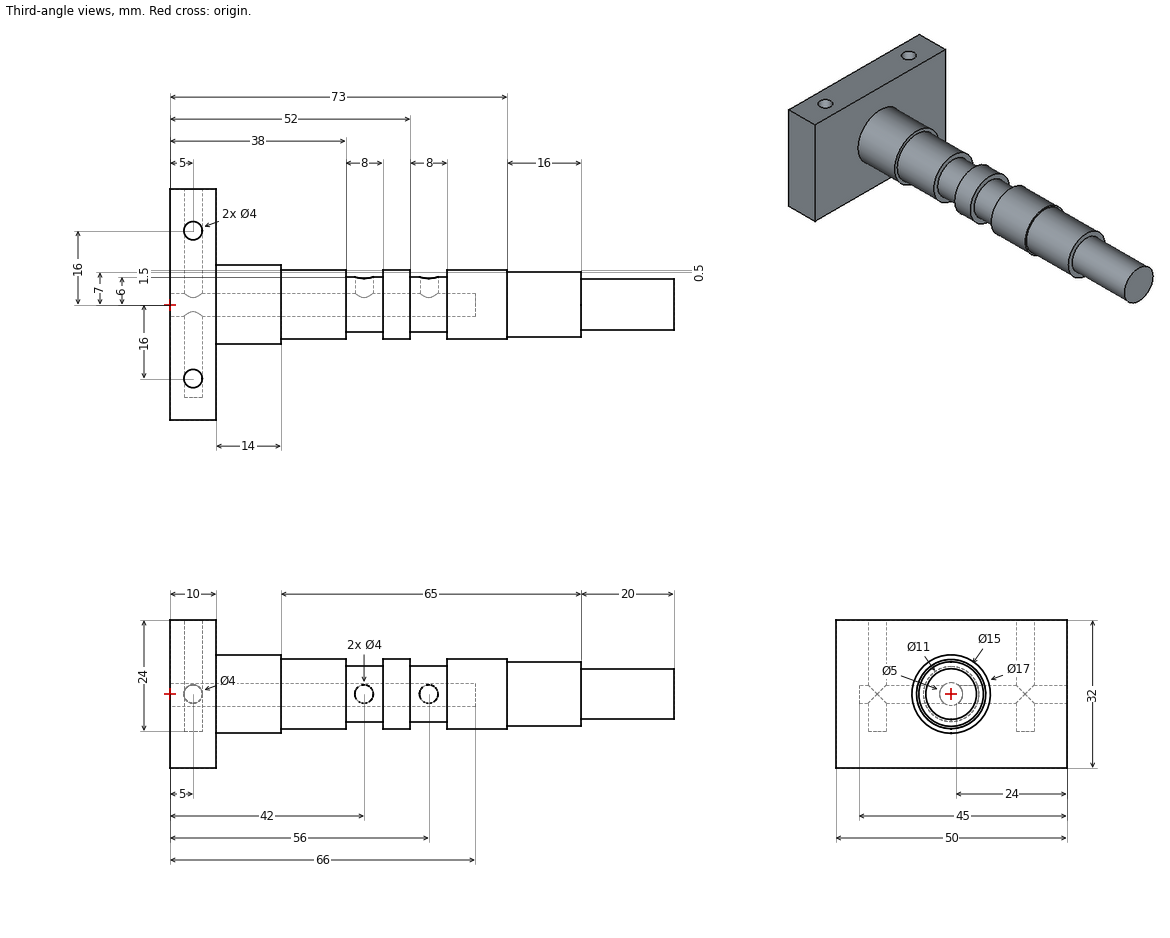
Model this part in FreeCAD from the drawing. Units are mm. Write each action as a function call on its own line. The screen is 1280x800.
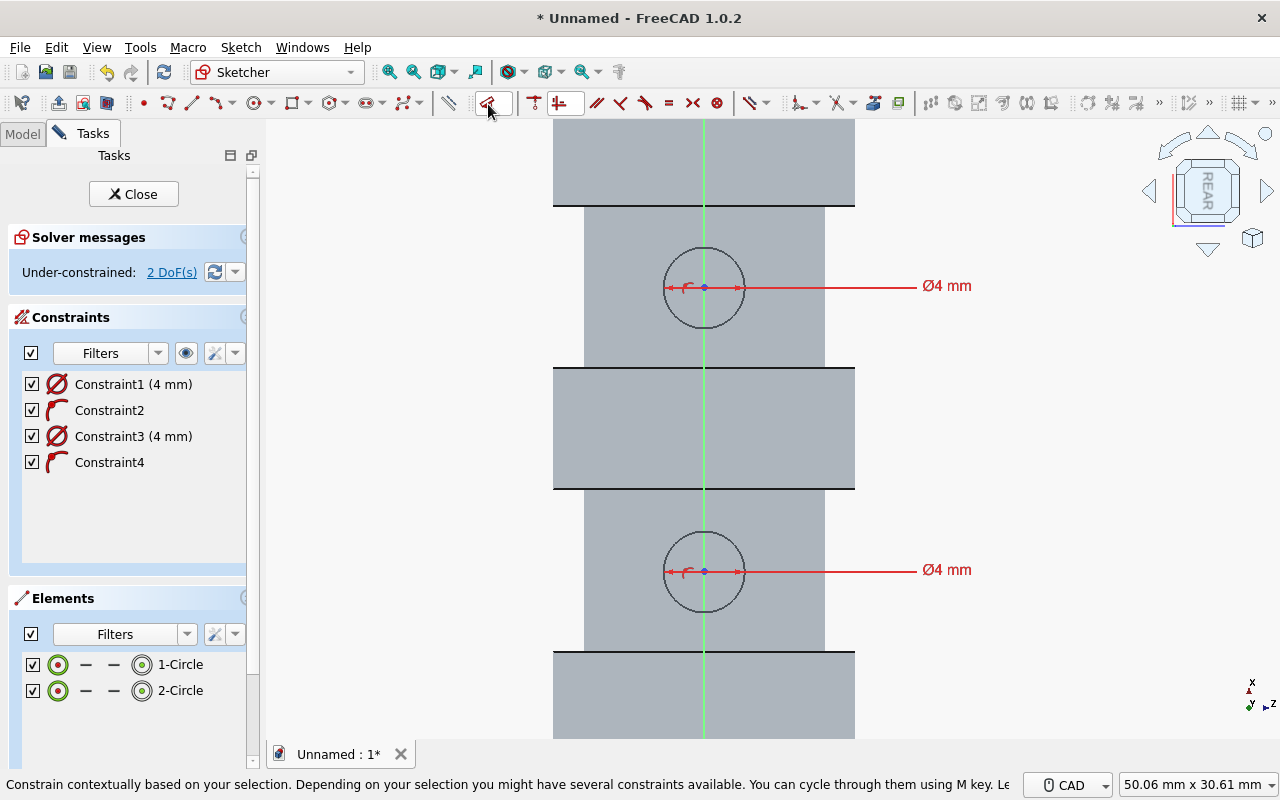
click(704, 572)
click(738, 642)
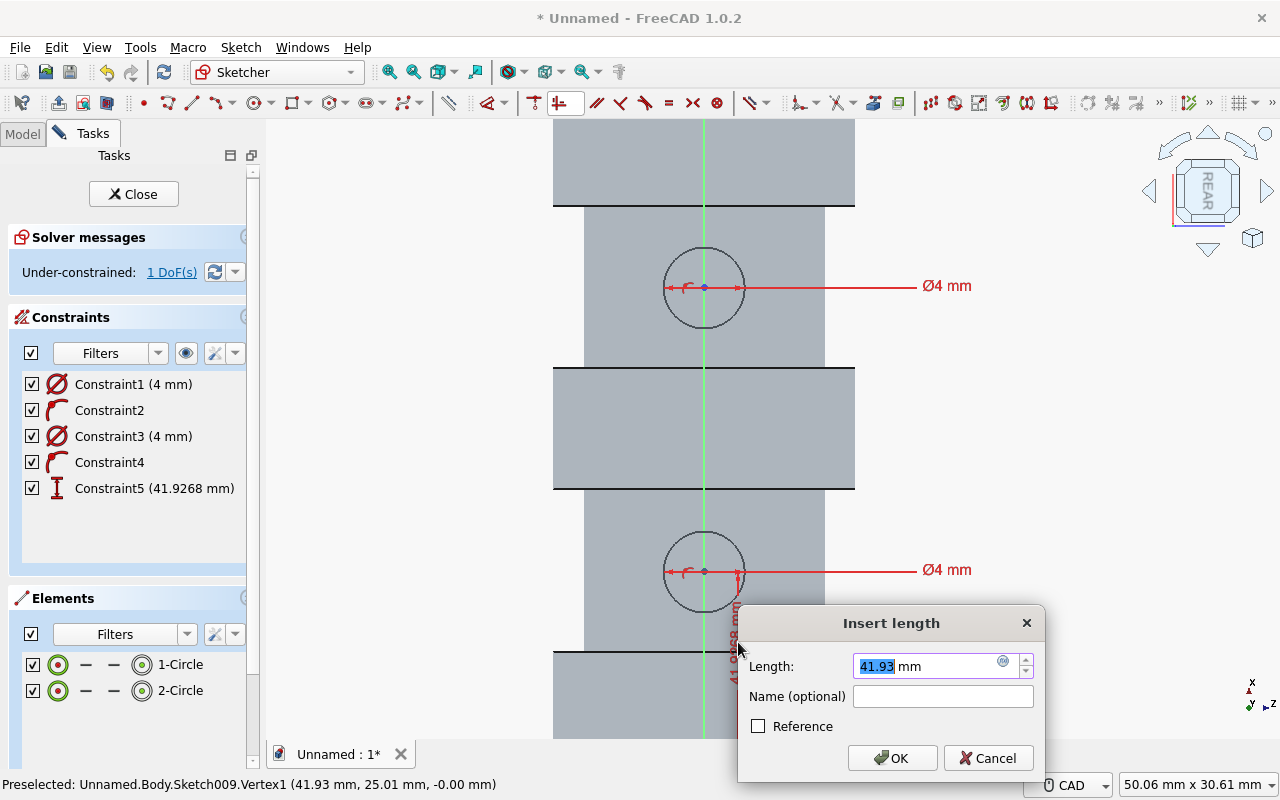
text(42)
key(Return)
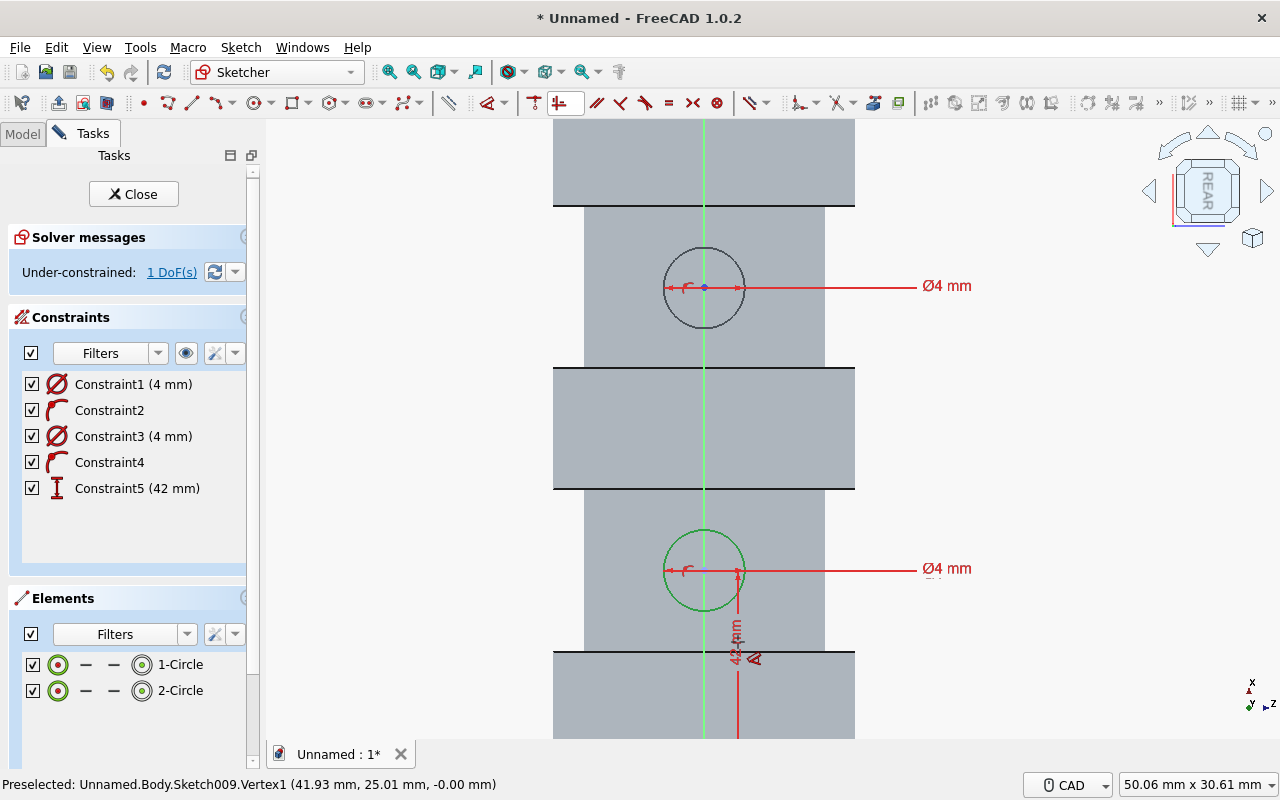
click(704, 288)
click(738, 499)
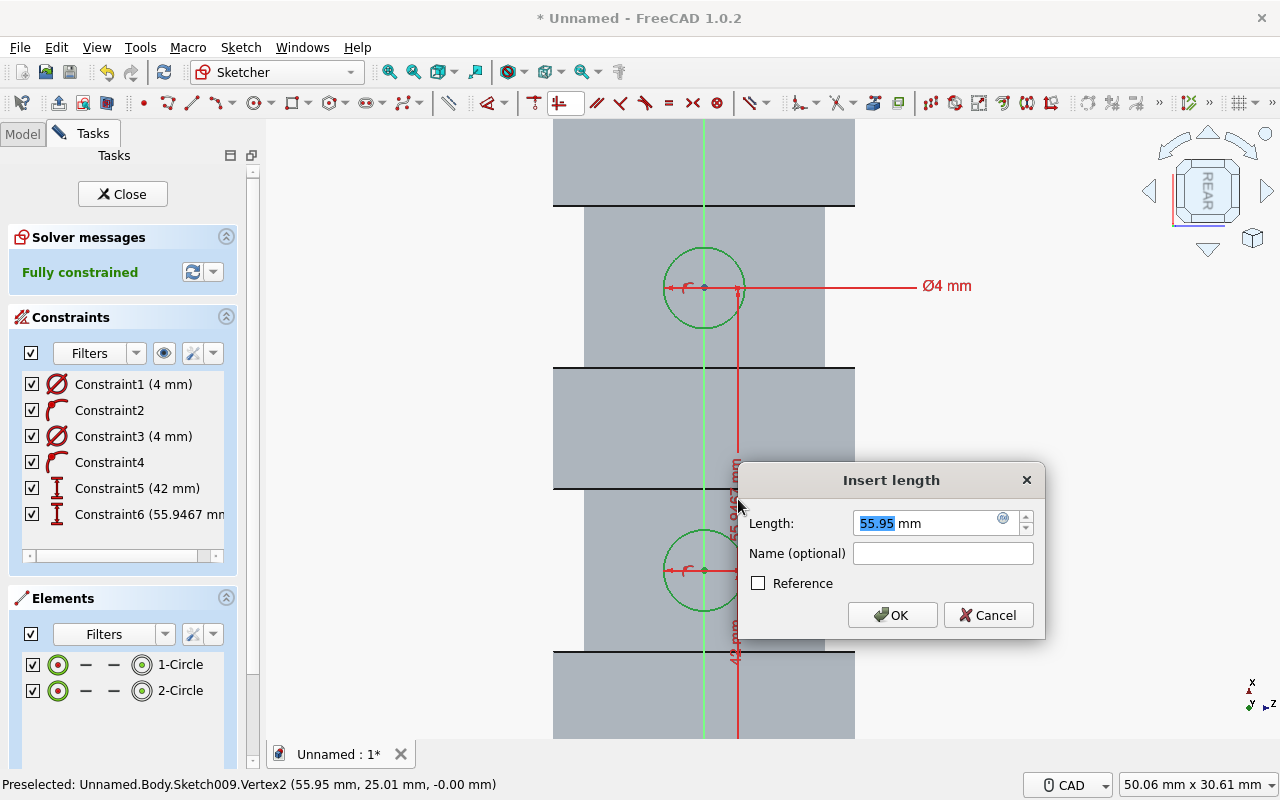
text(56)
key(Return)
key(Escape)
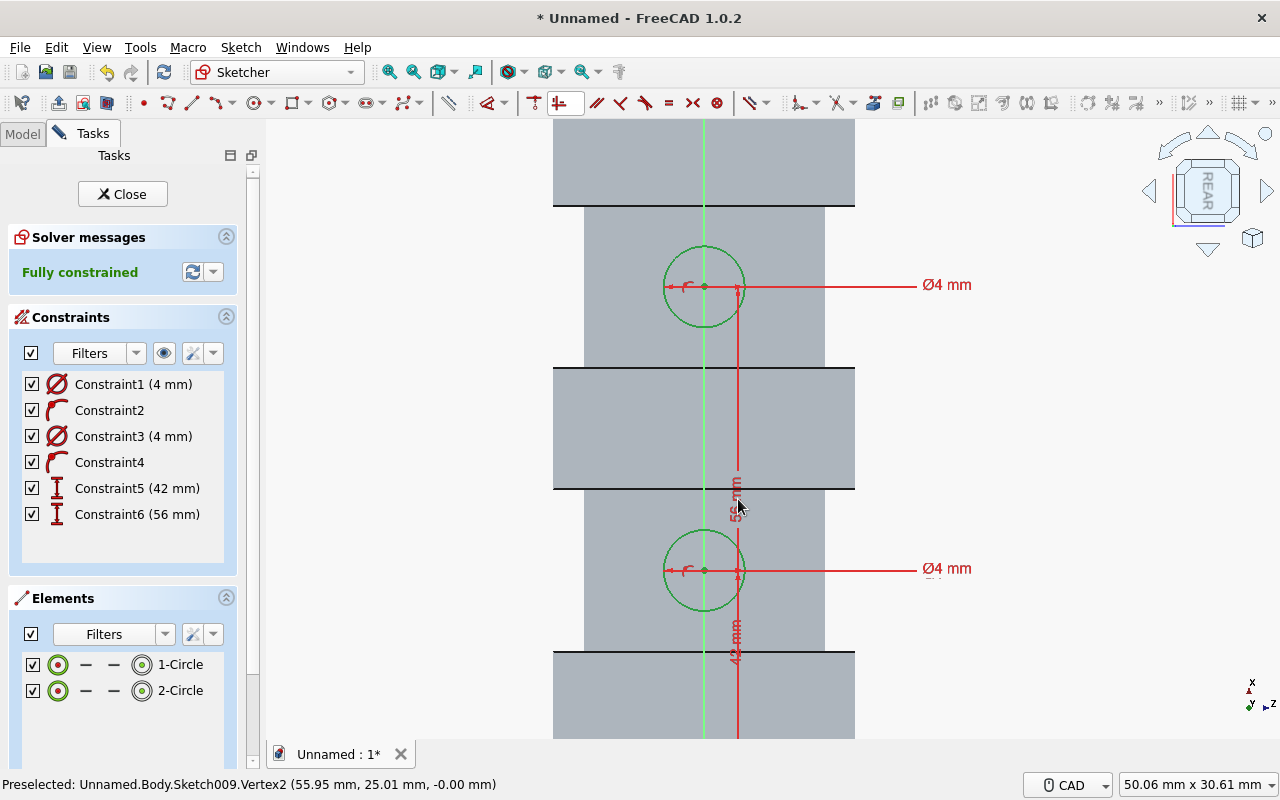
click(123, 194)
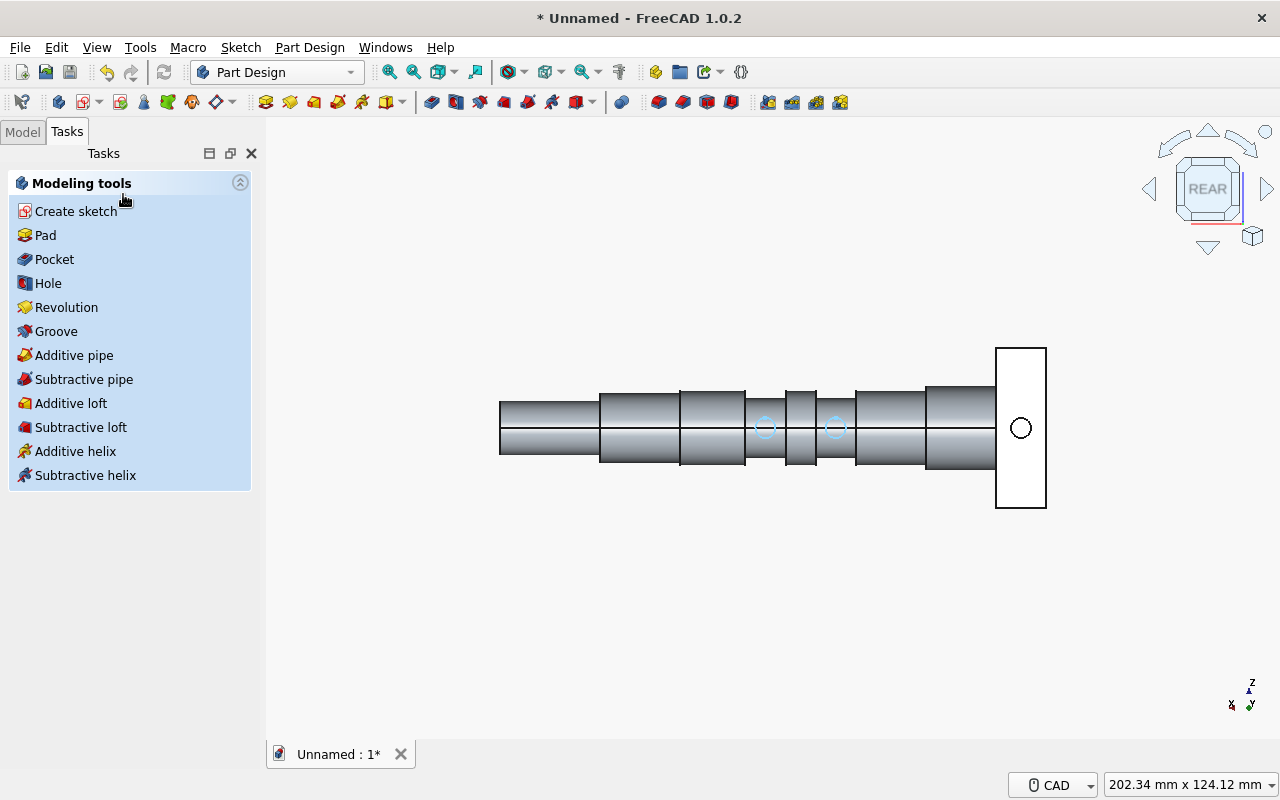
click(432, 102)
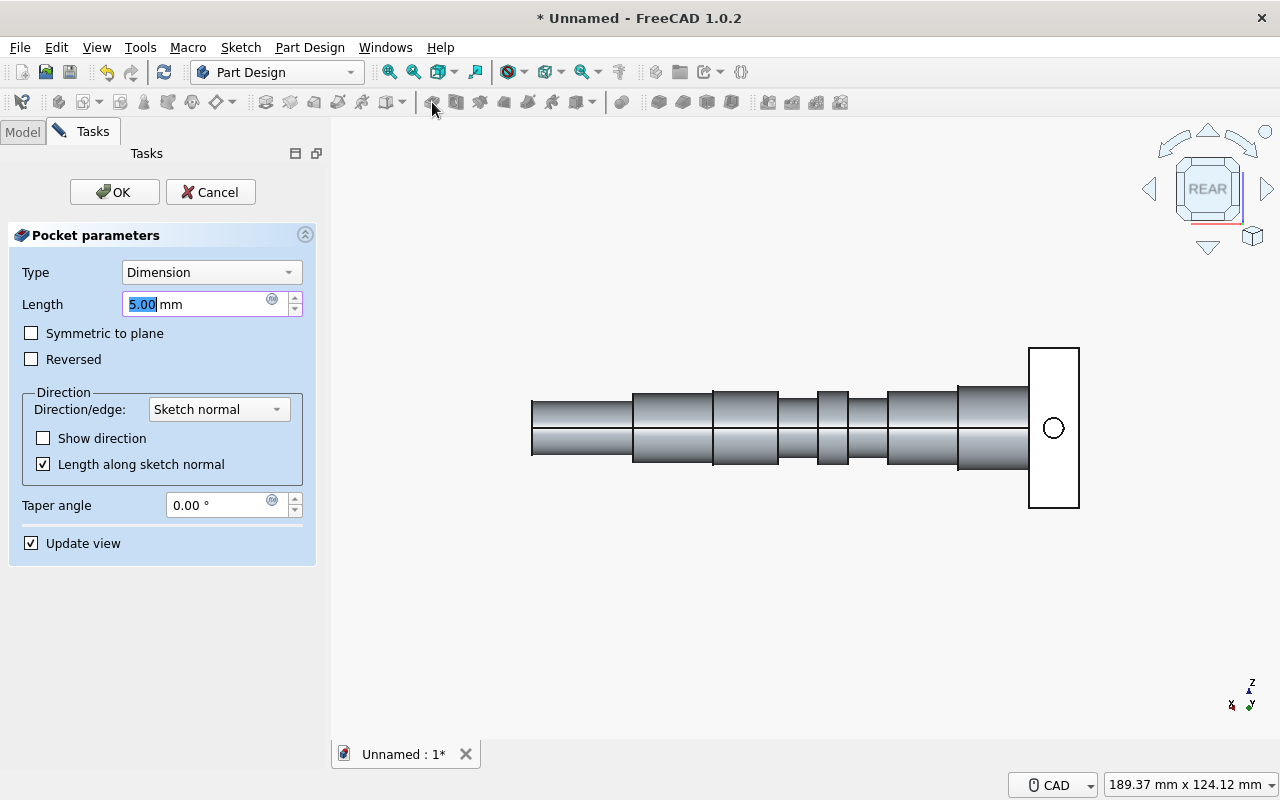
text(24)
key(Tab)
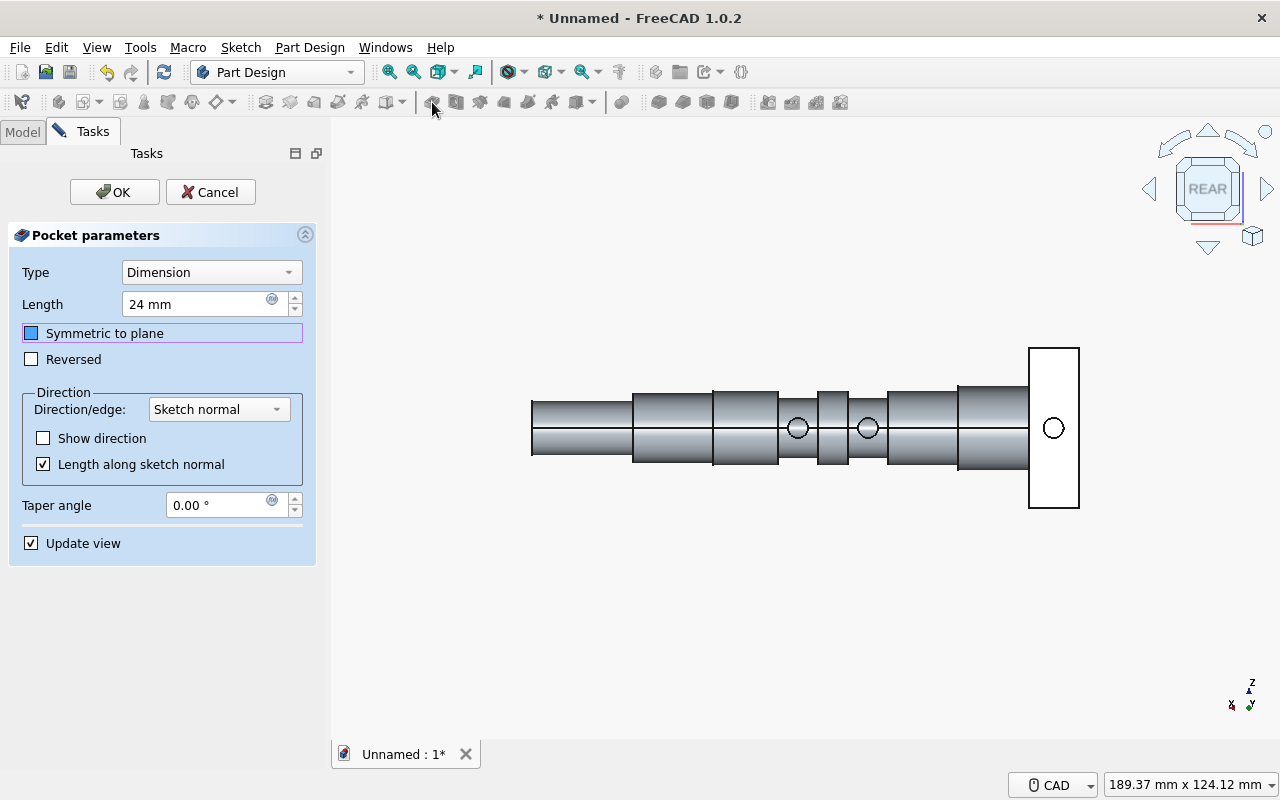
click(115, 192)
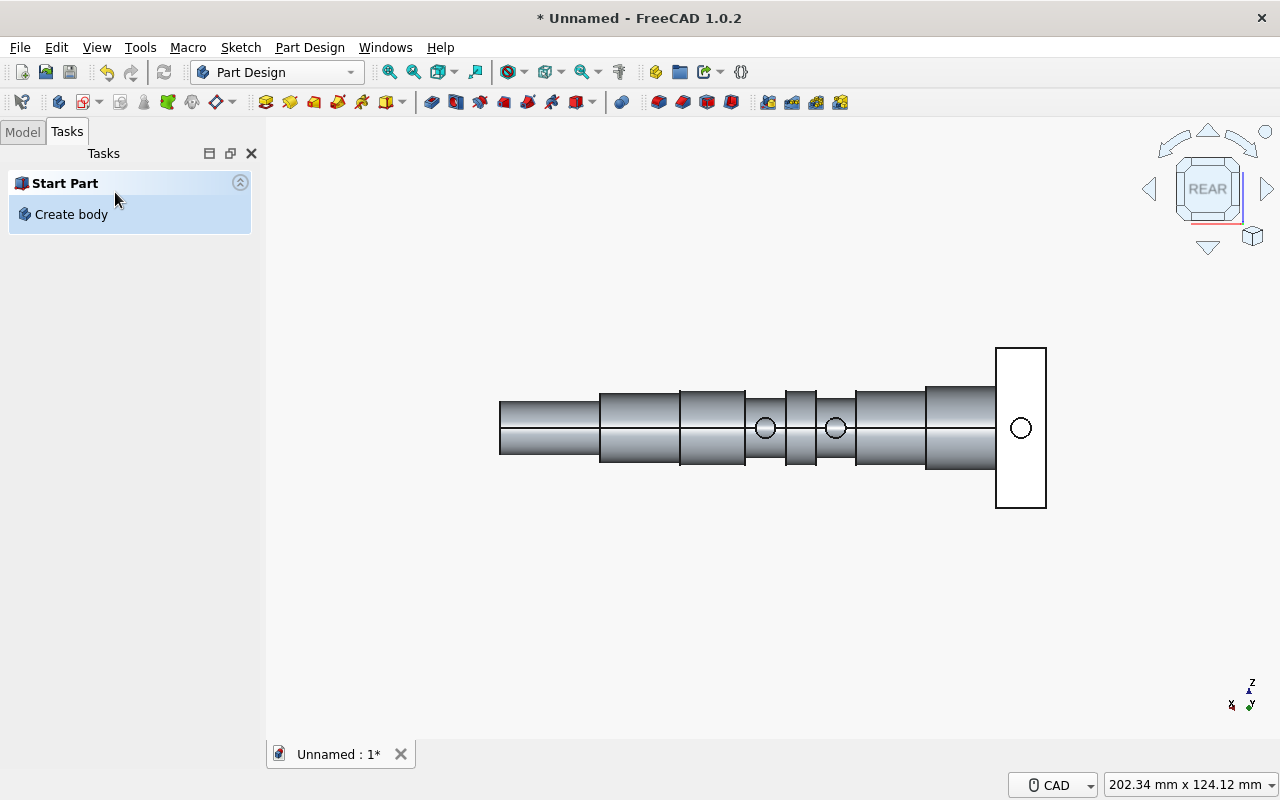
key(0)